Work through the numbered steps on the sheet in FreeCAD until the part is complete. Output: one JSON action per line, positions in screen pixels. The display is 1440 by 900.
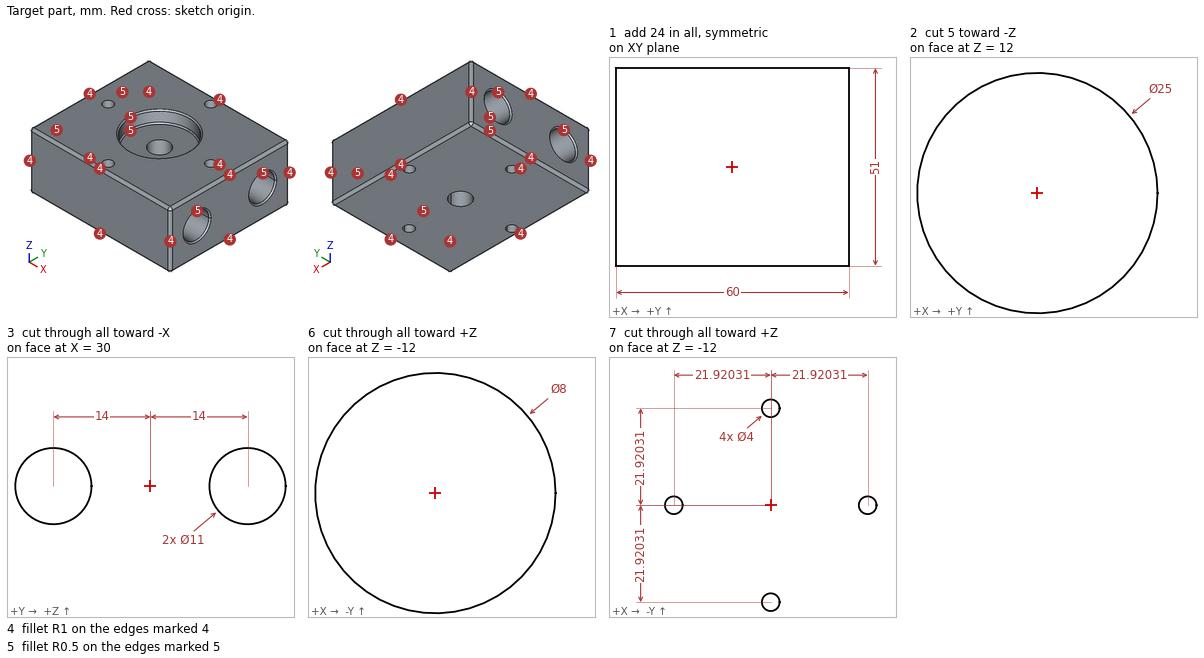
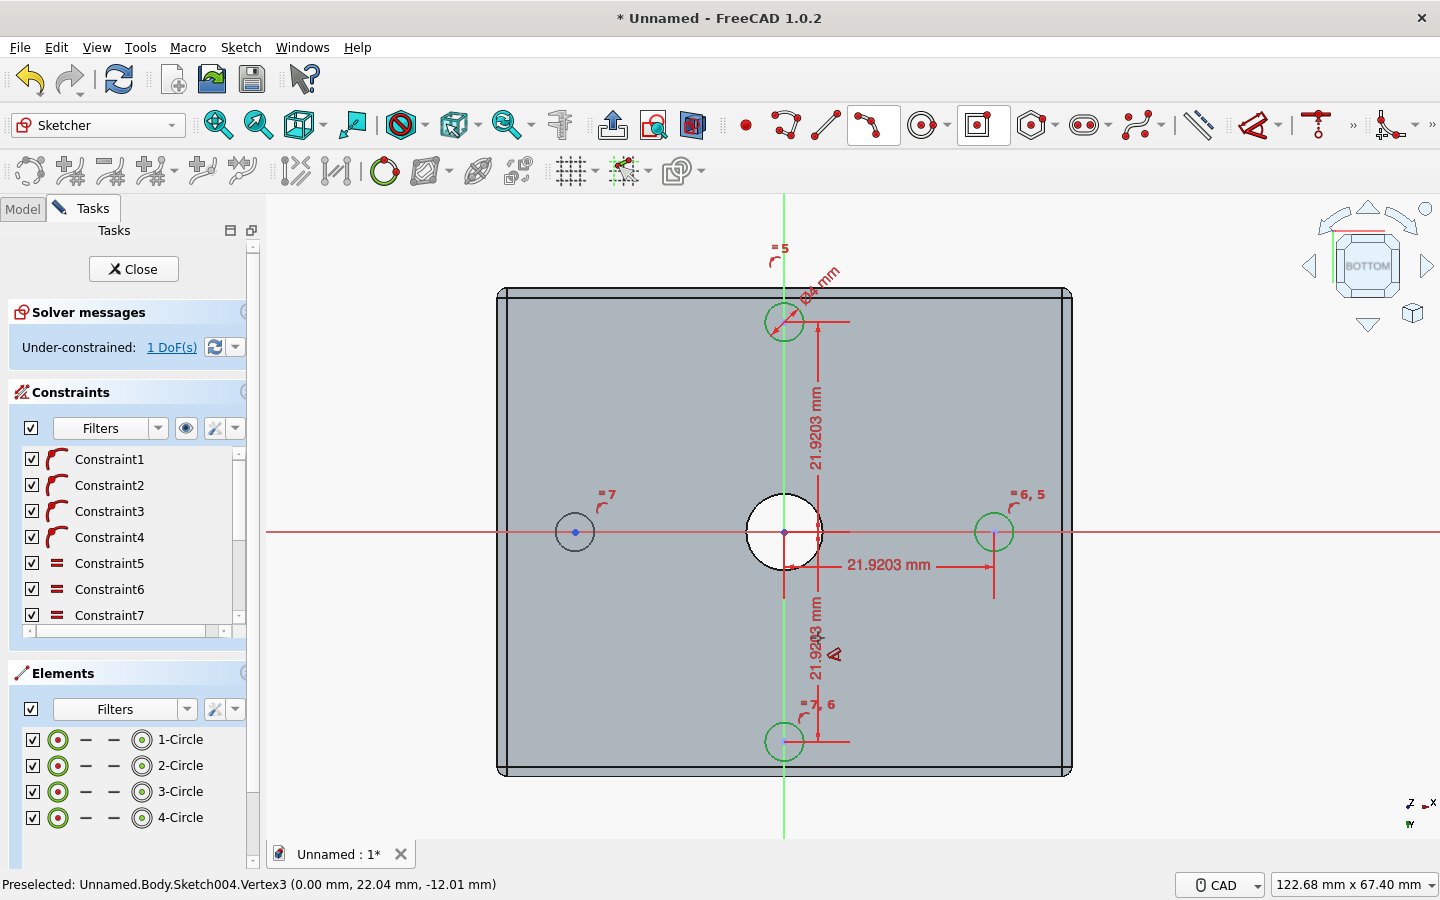
{"action": "left_click", "coordinate": [575, 532]}
{"action": "left_click", "coordinate": [680, 566]}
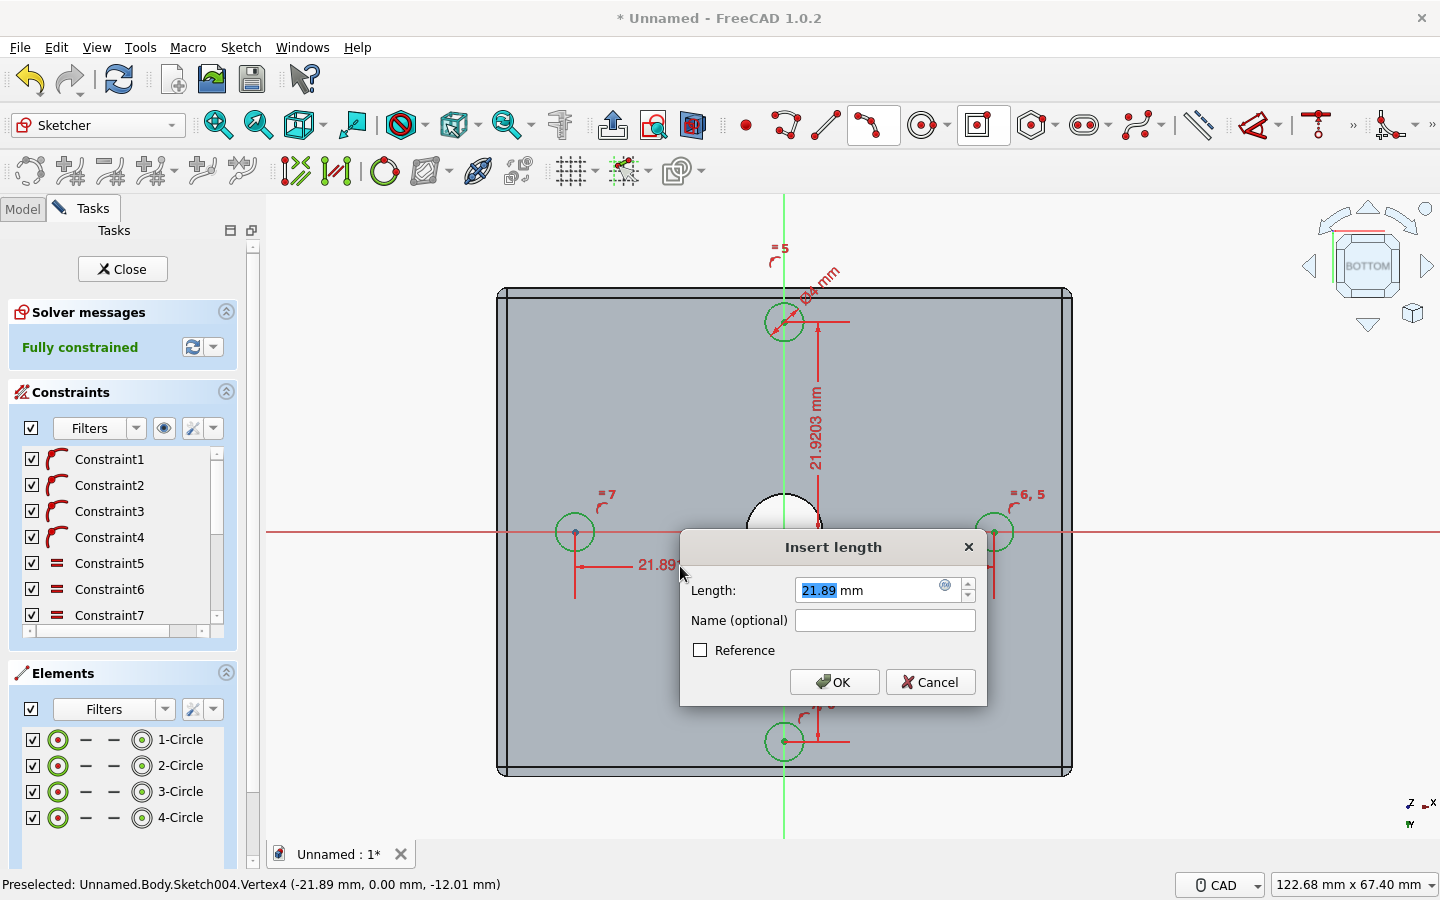
{"action": "type", "text": "21.92031"}
{"action": "key", "text": "Return"}
{"action": "key", "text": "Escape"}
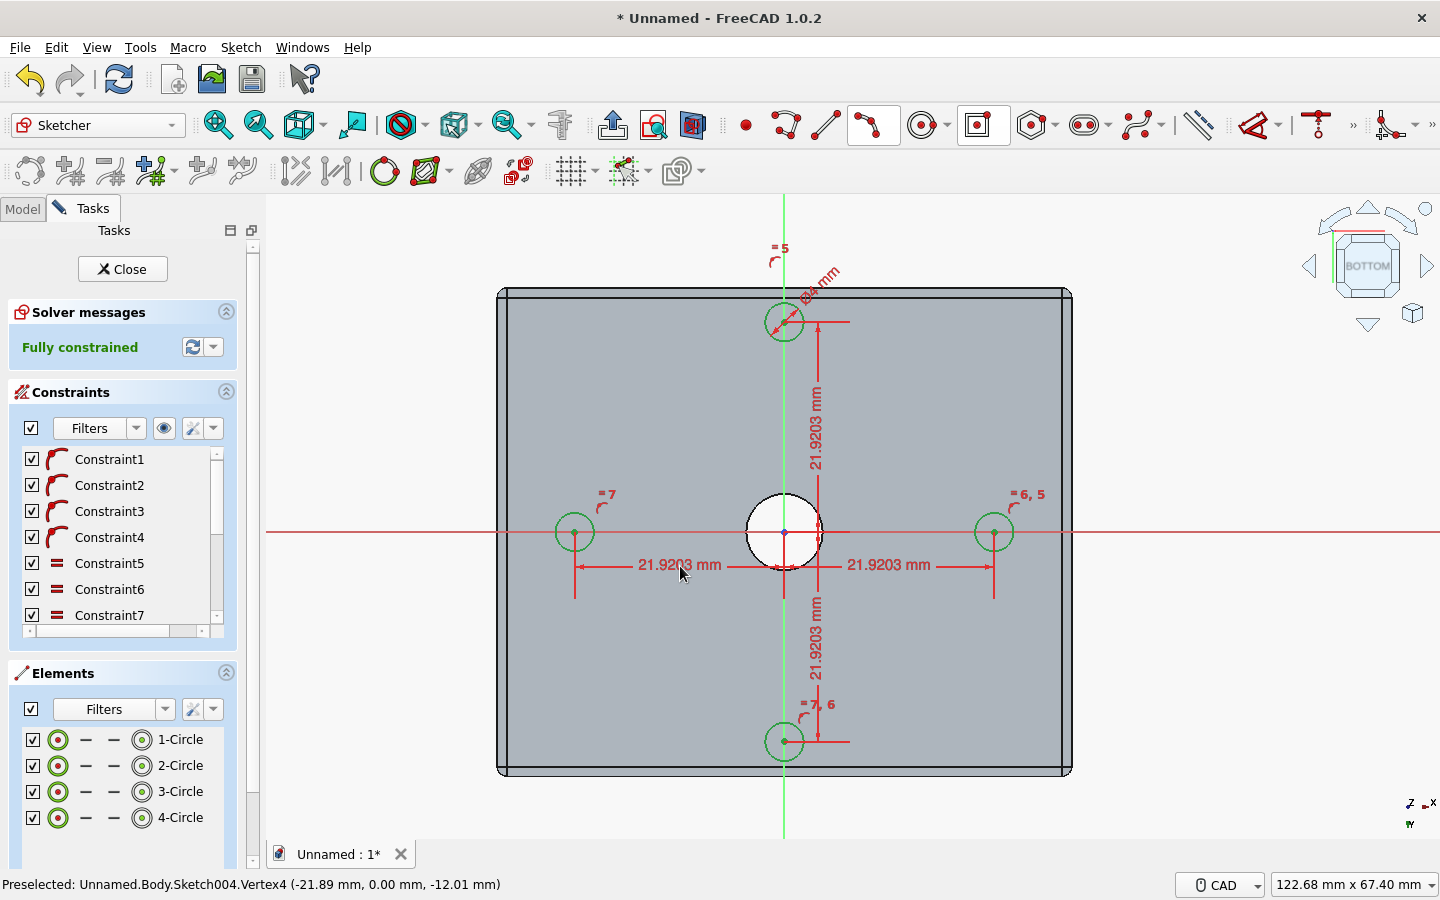
{"action": "left_click", "coordinate": [123, 269]}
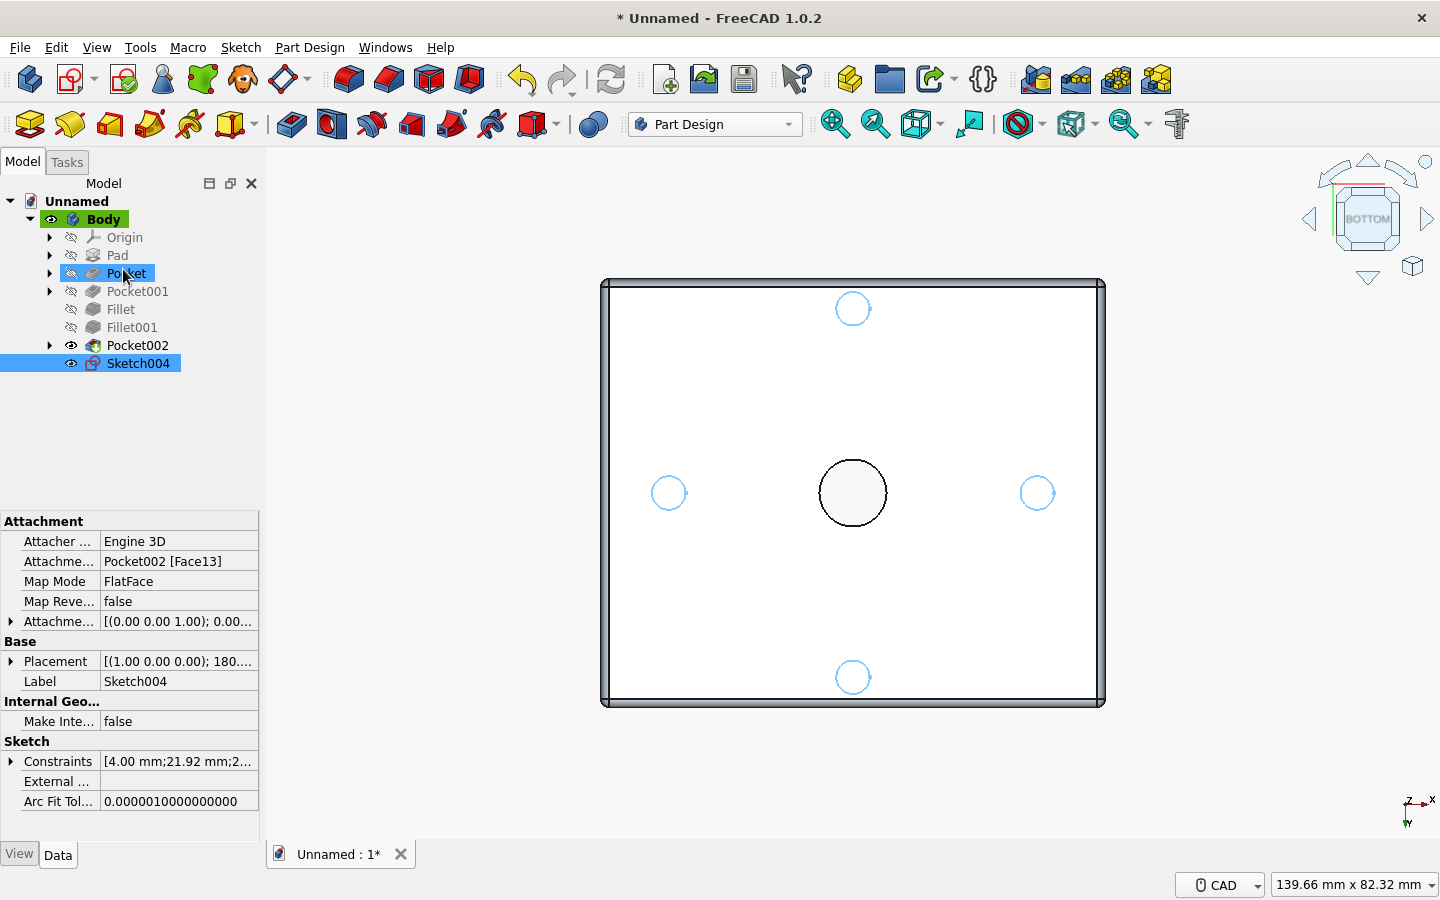
{"action": "left_click", "coordinate": [292, 124]}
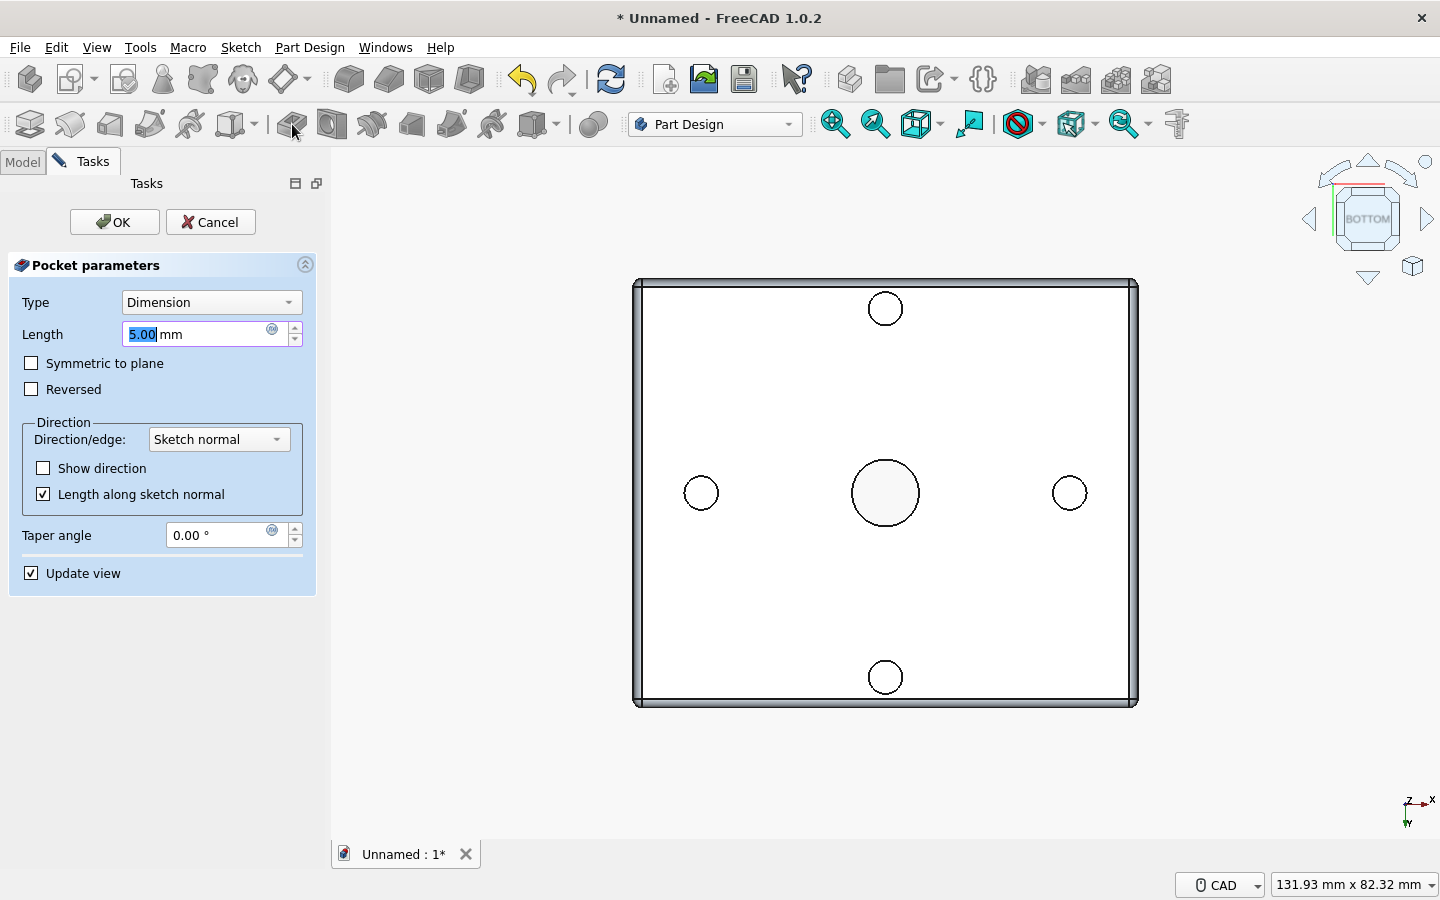
{"action": "left_click", "coordinate": [212, 302]}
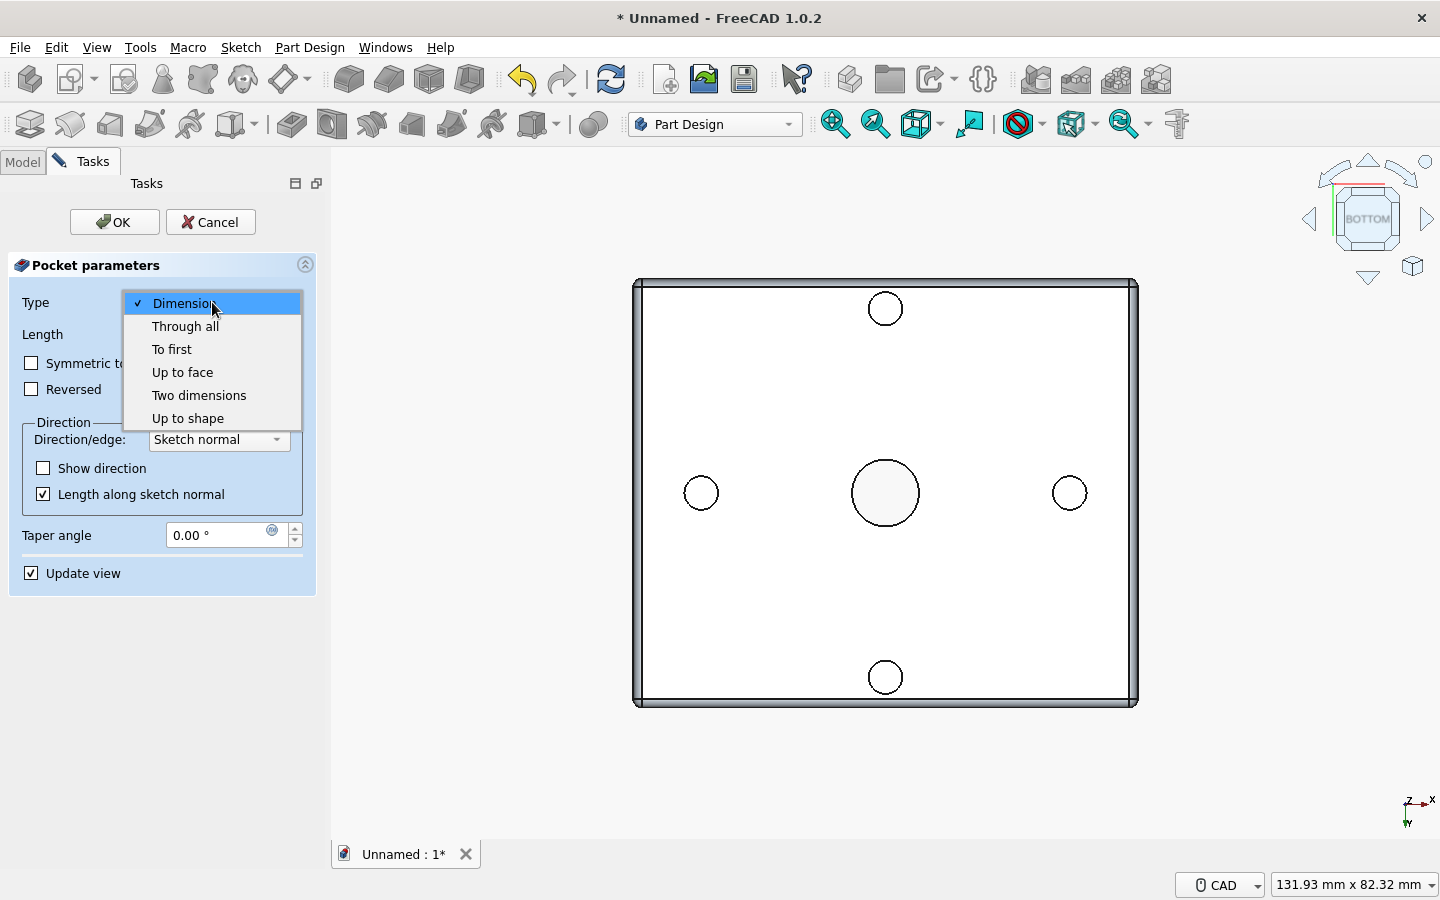
{"action": "left_click", "coordinate": [212, 326]}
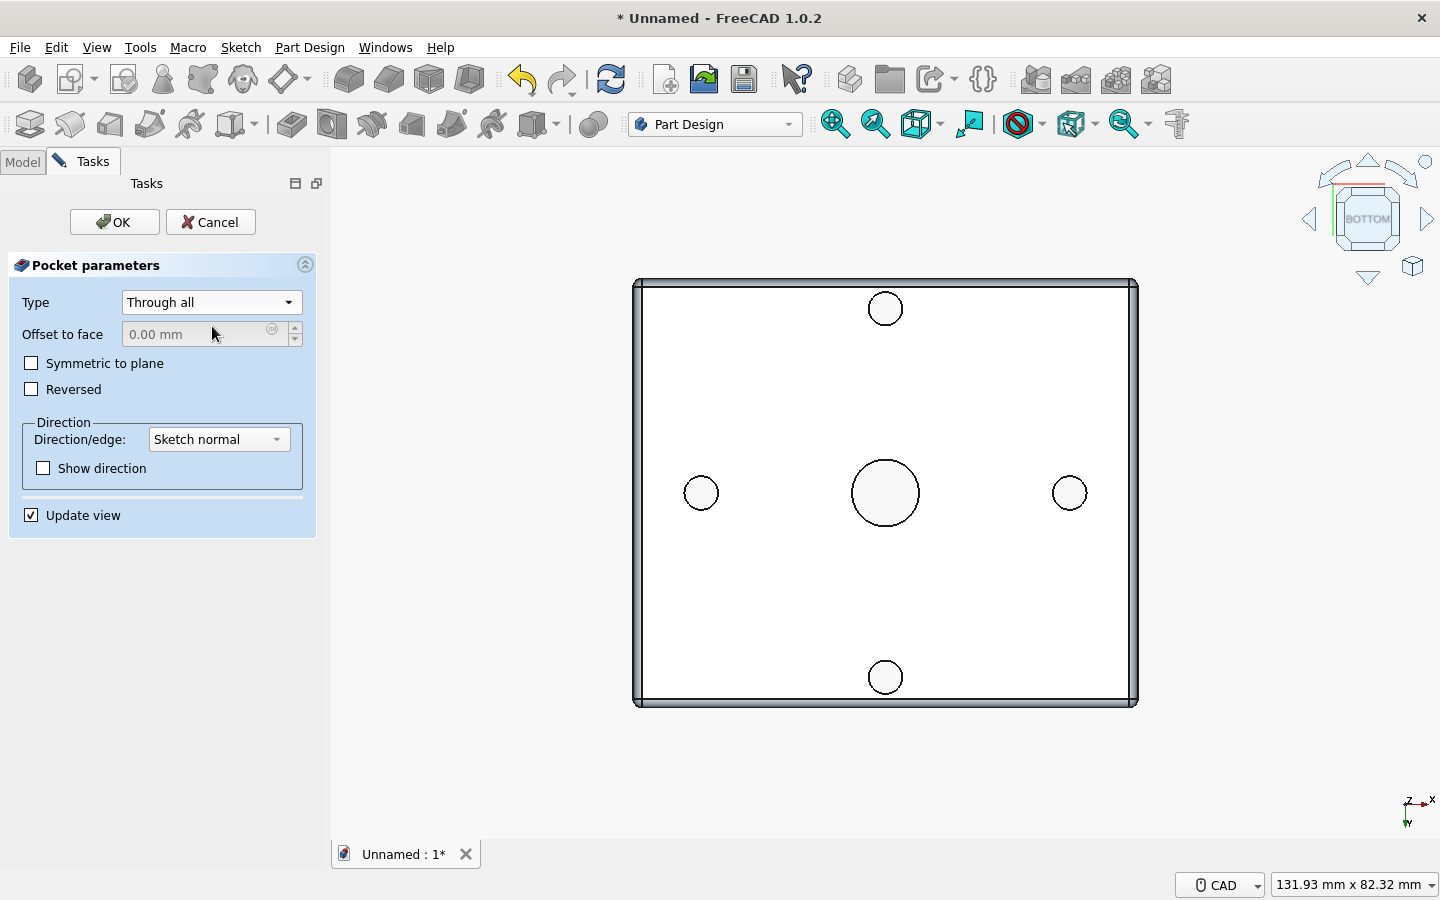
{"action": "left_click", "coordinate": [115, 222]}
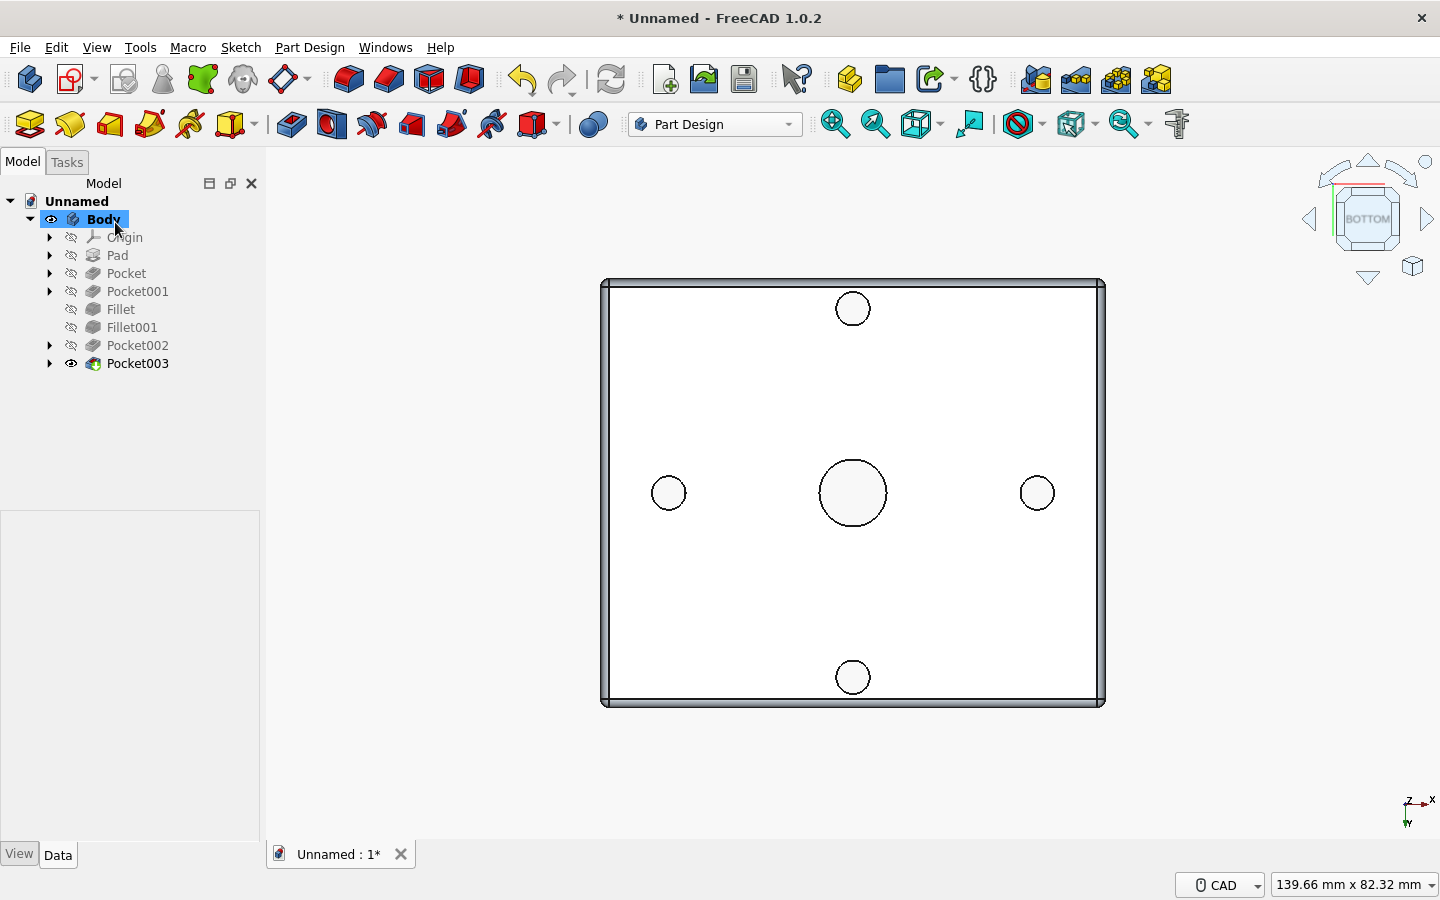
{"action": "key", "text": "0"}